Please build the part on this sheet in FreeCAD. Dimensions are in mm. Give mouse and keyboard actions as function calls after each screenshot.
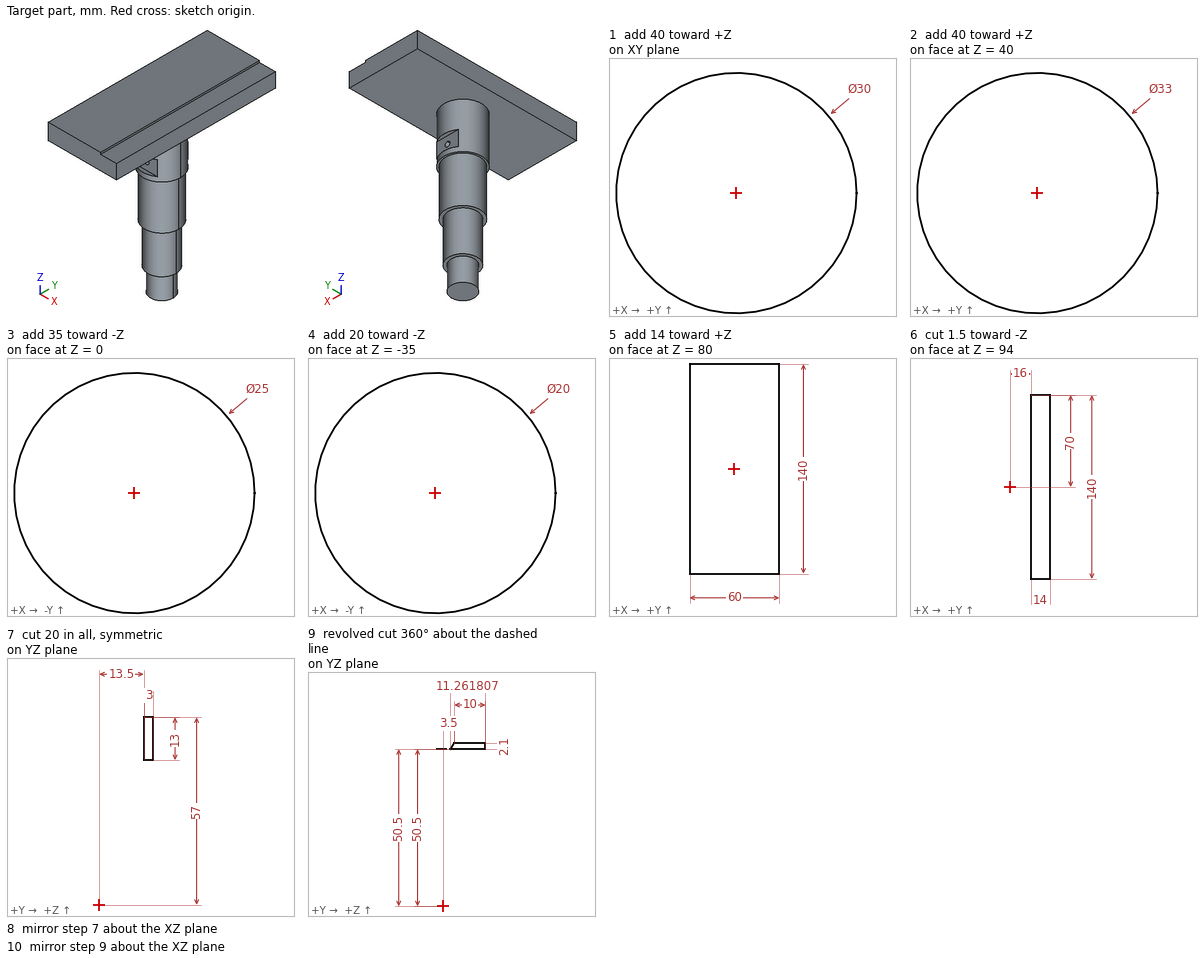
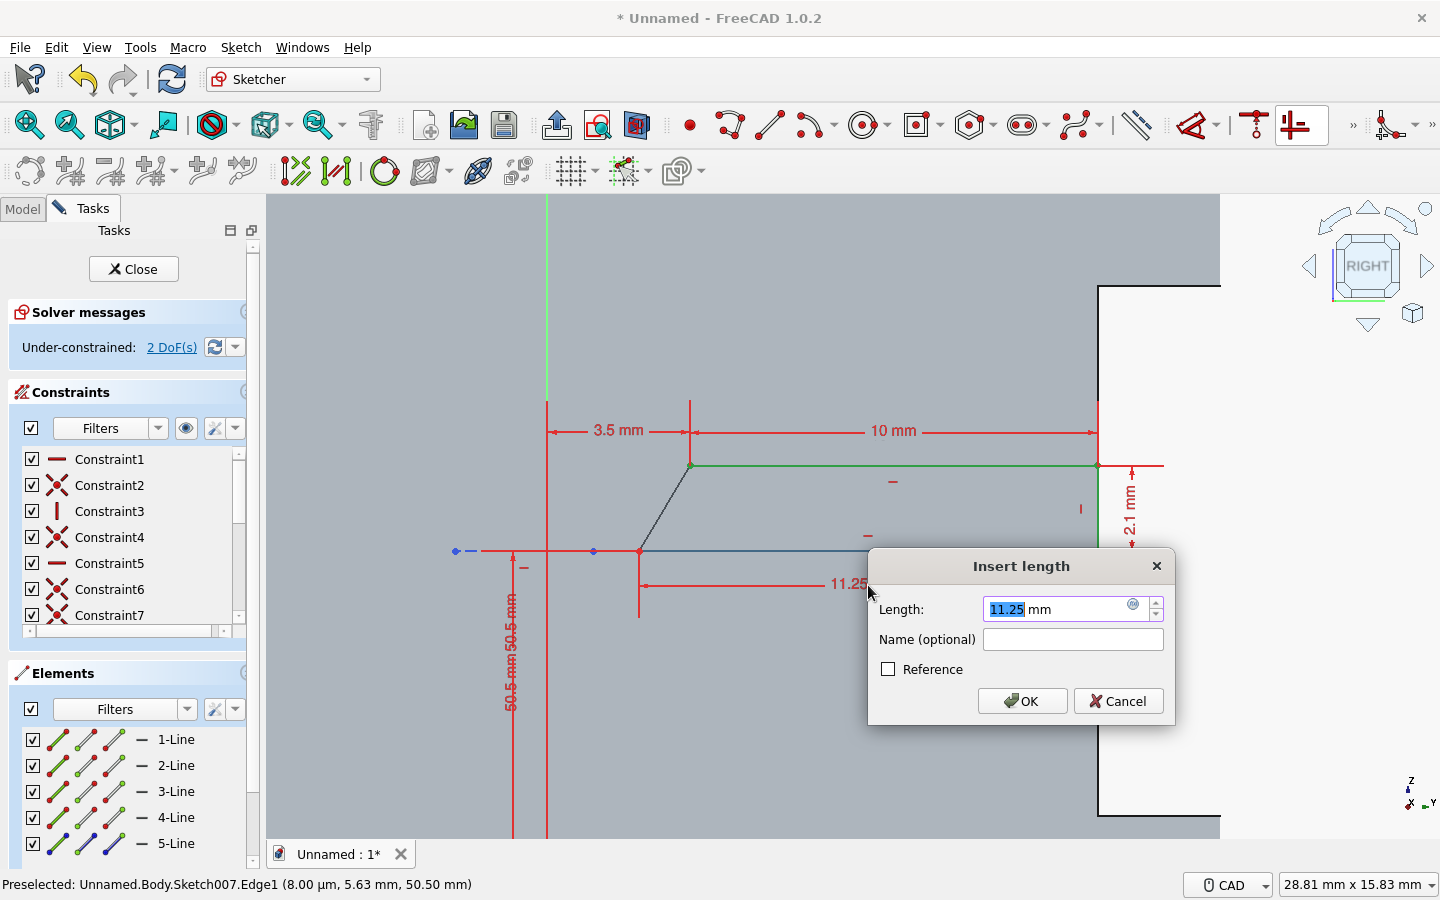
text(11.261807)
key(Return)
key(Escape)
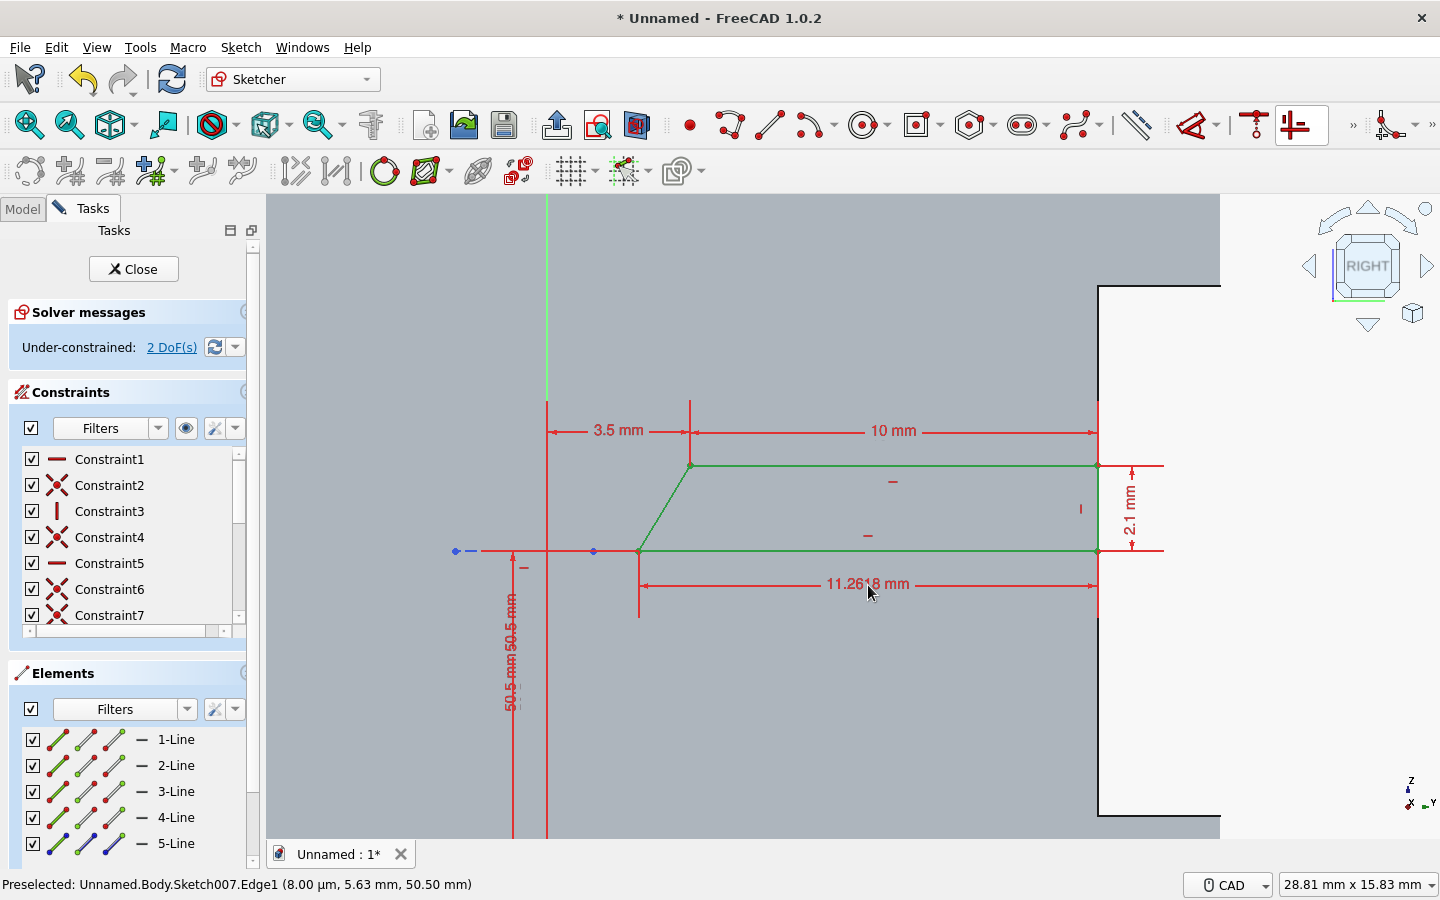
click(134, 269)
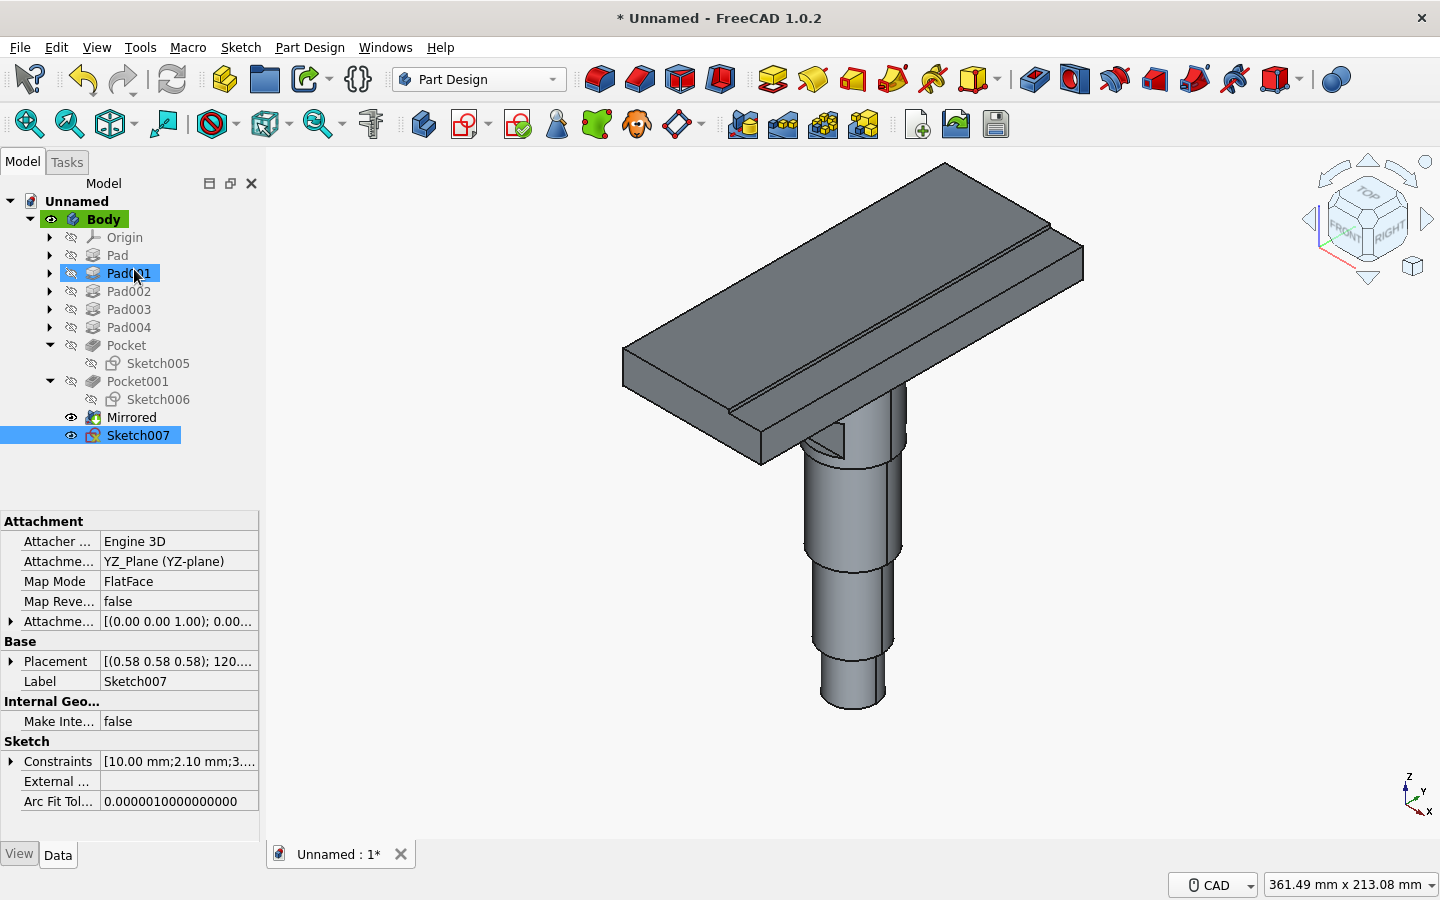
click(1116, 80)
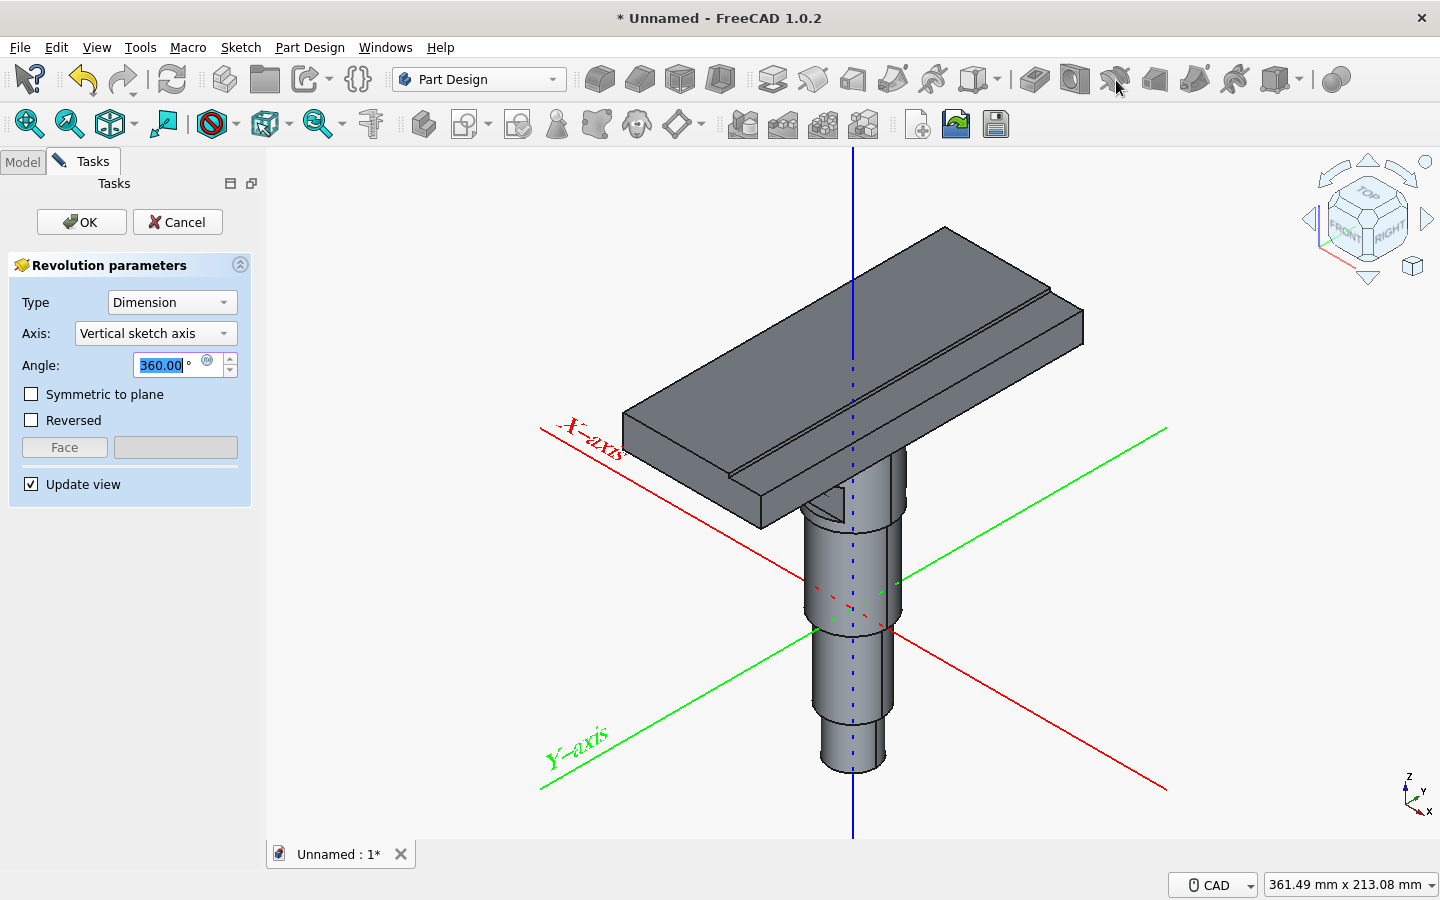
click(156, 334)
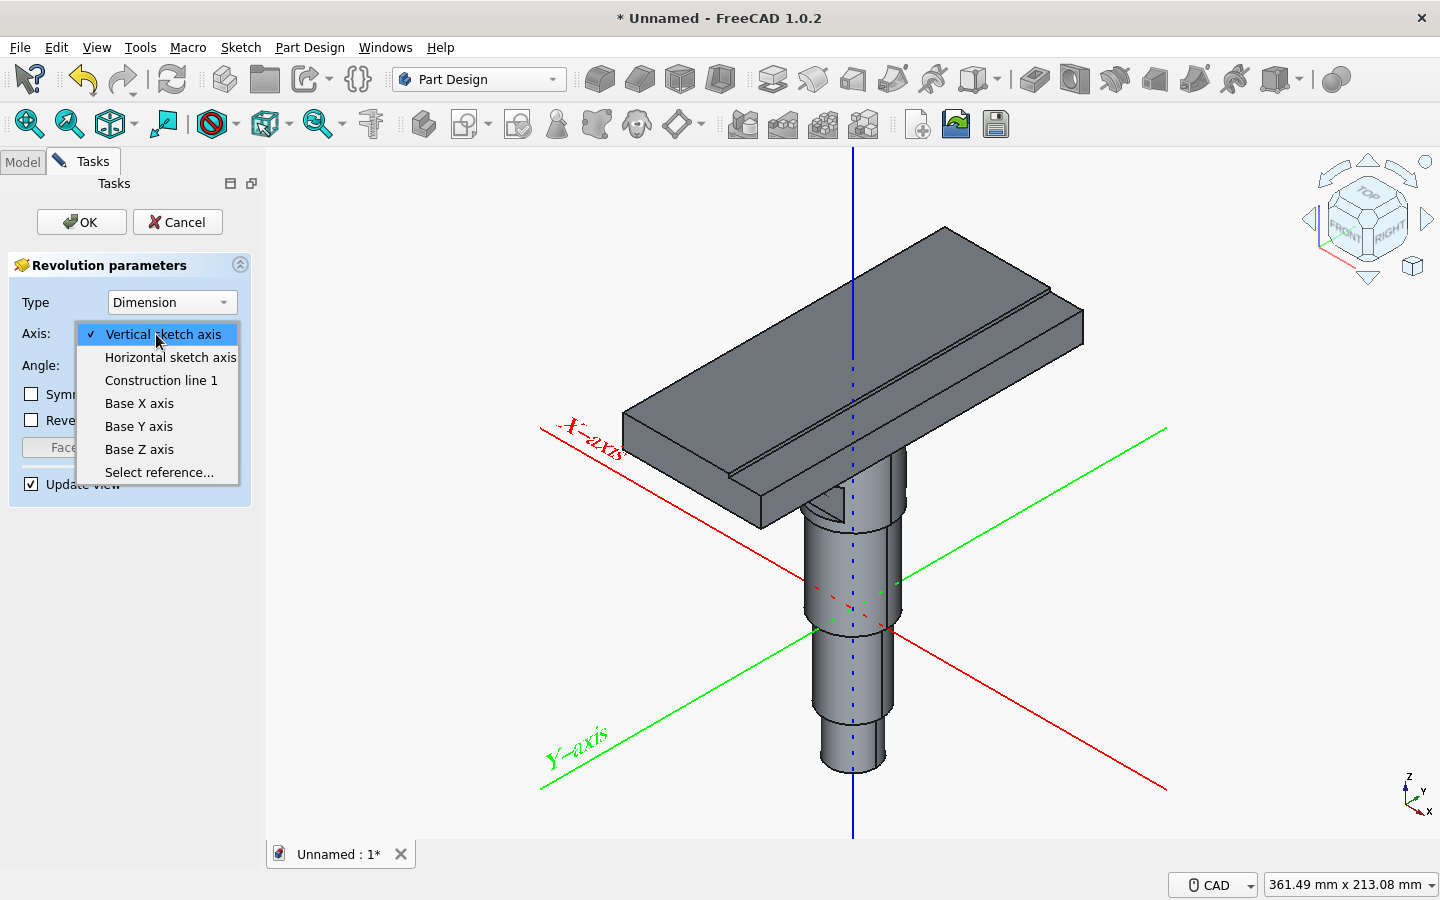
click(156, 380)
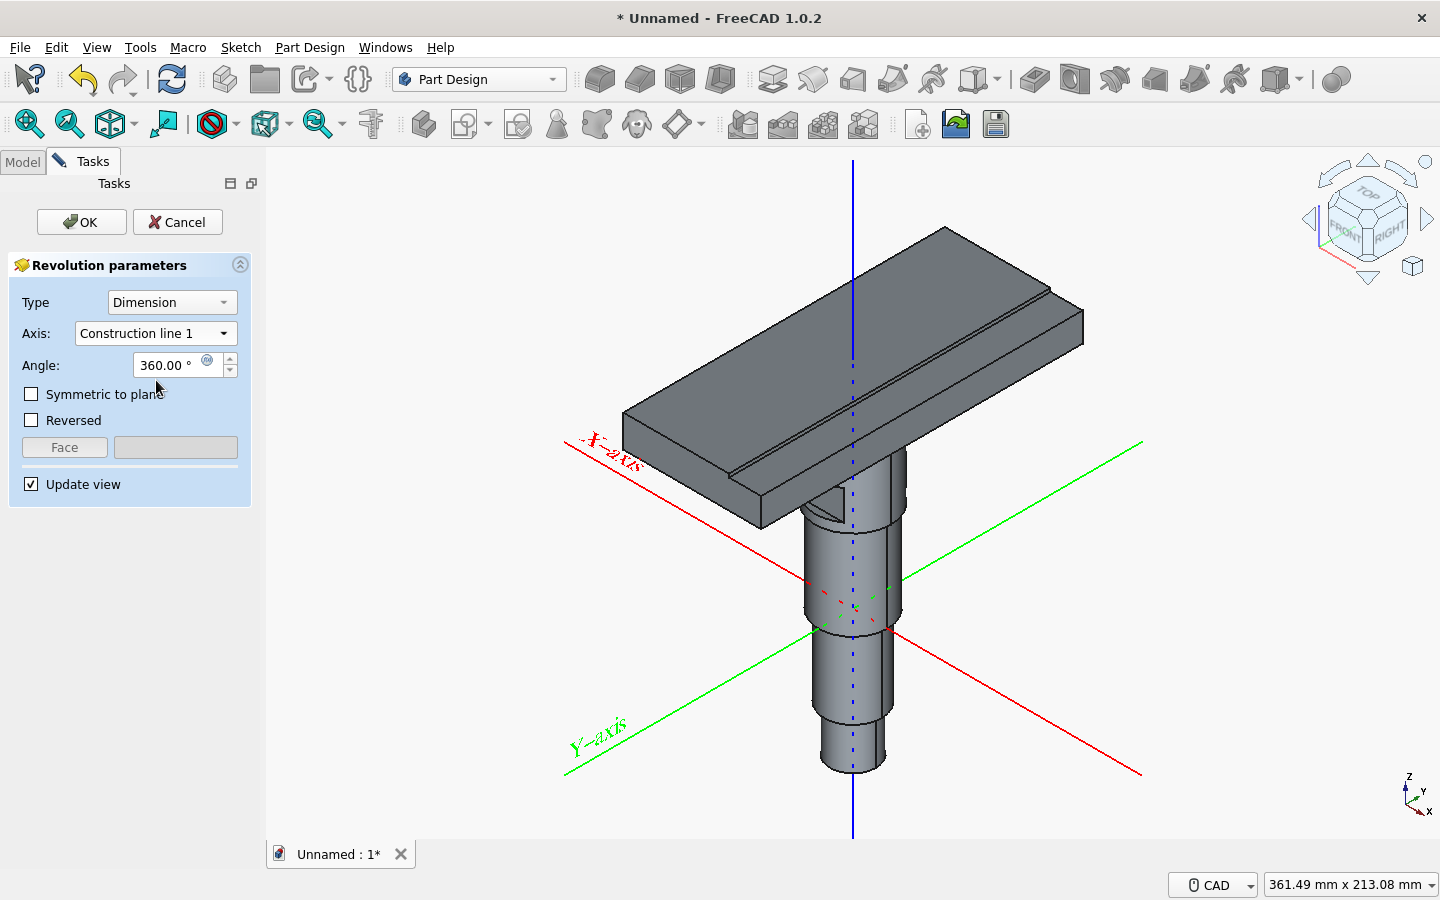
click(82, 222)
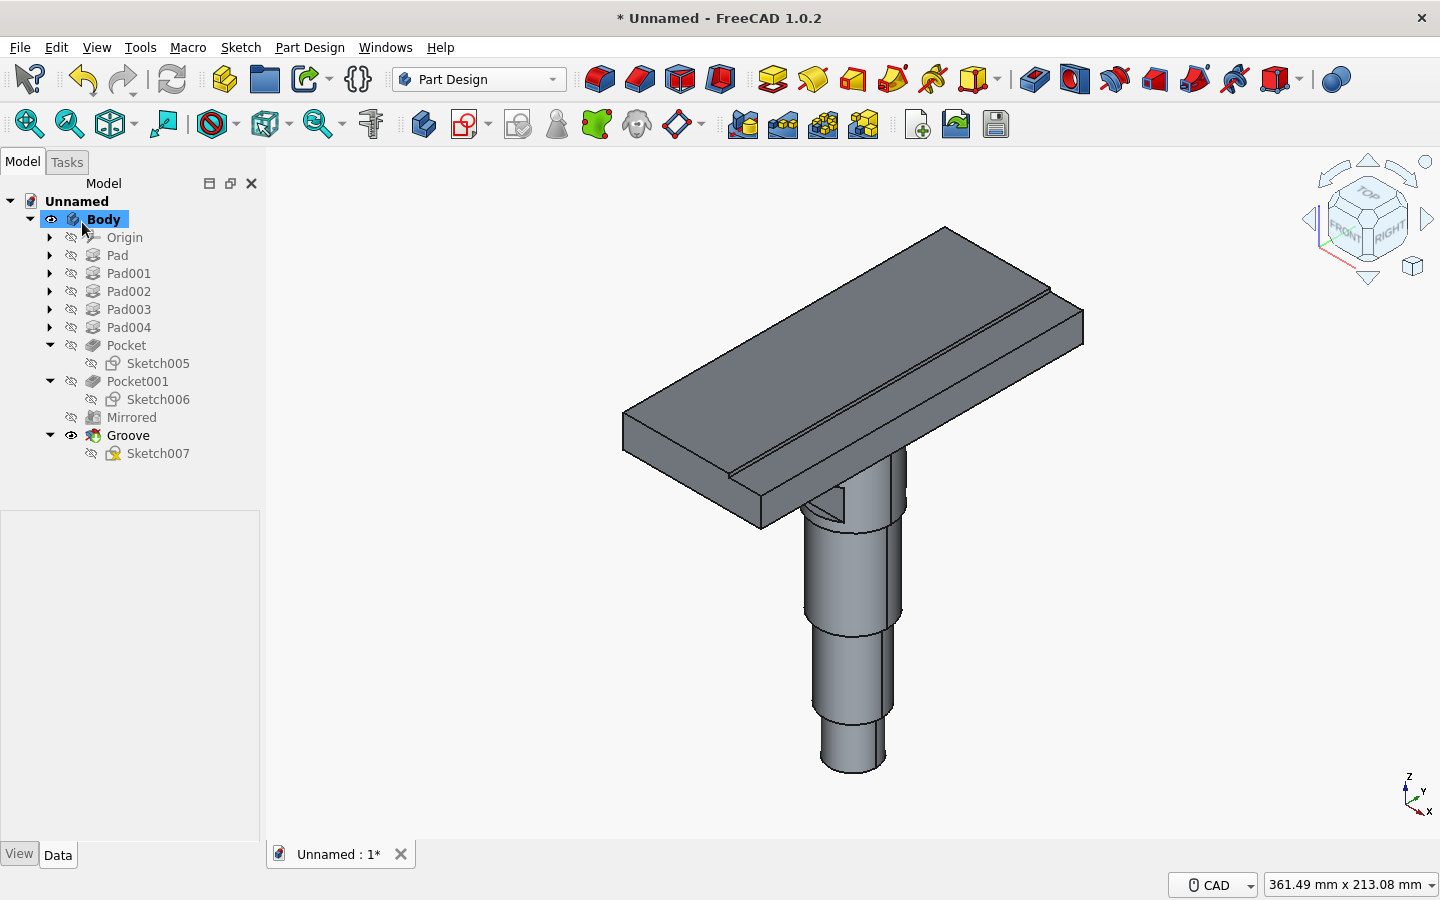
click(30, 124)